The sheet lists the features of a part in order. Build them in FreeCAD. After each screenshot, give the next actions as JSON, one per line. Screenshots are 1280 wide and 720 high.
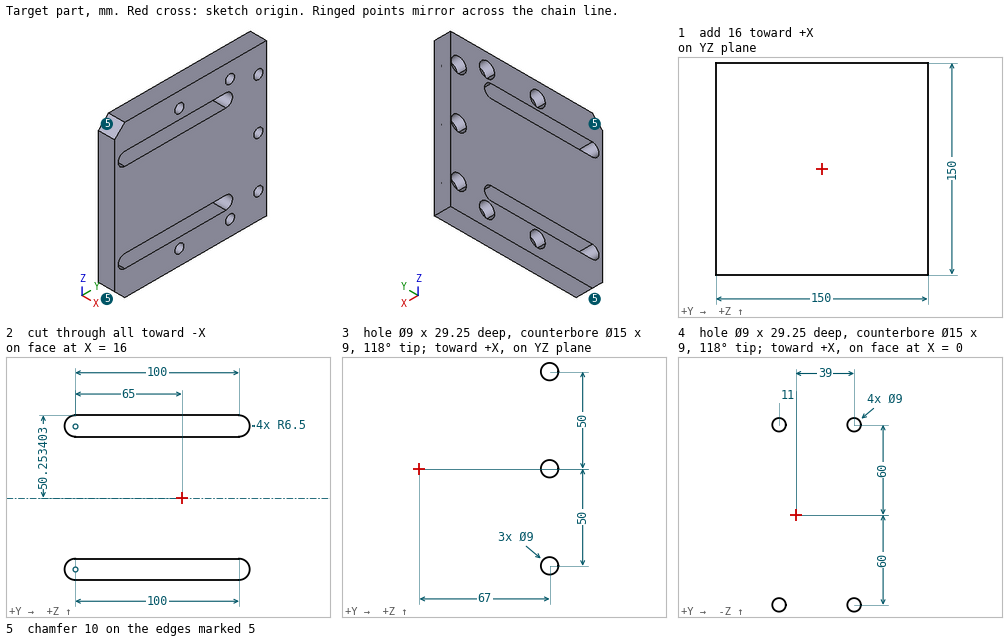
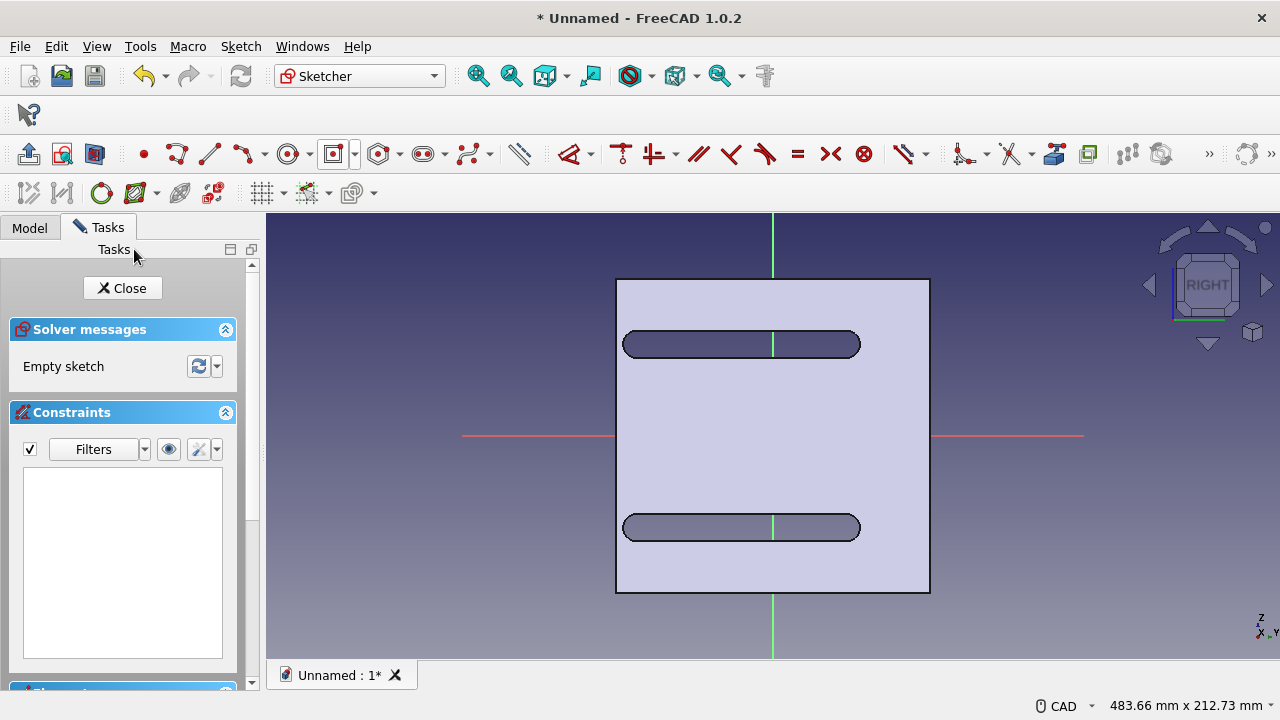
{"action": "left_click", "coordinate": [95, 154]}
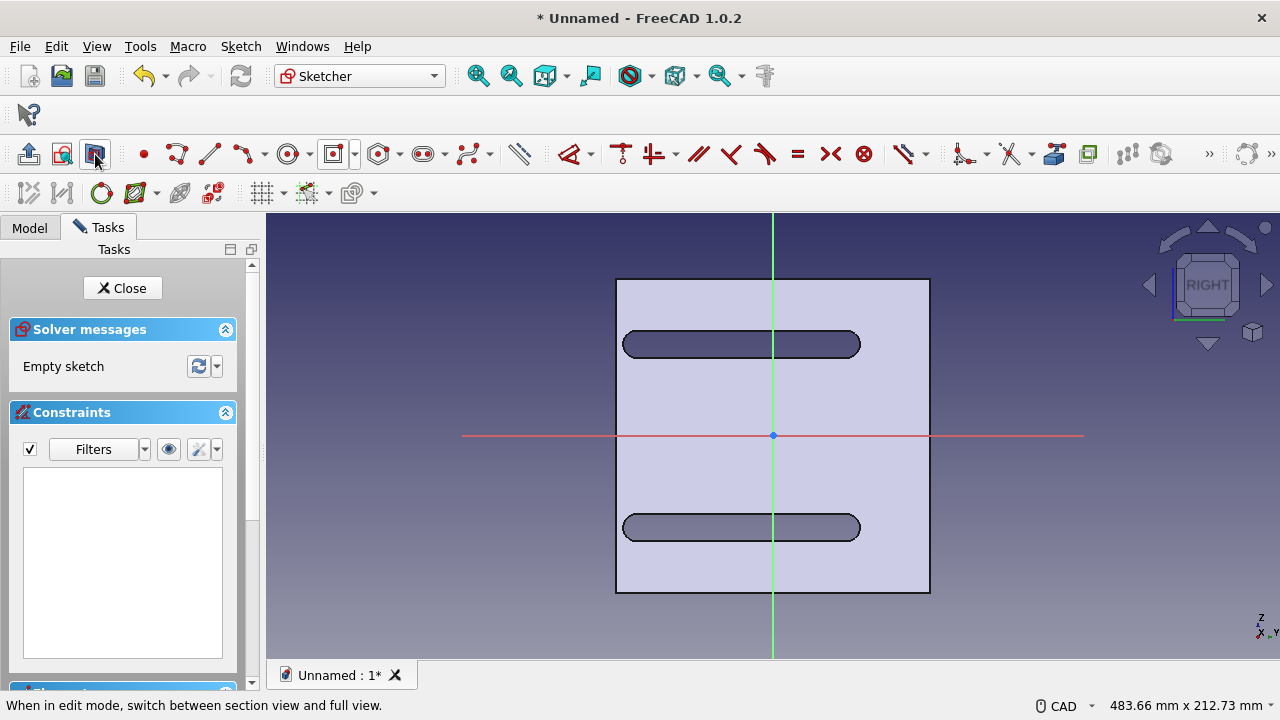
{"action": "key", "text": "g c"}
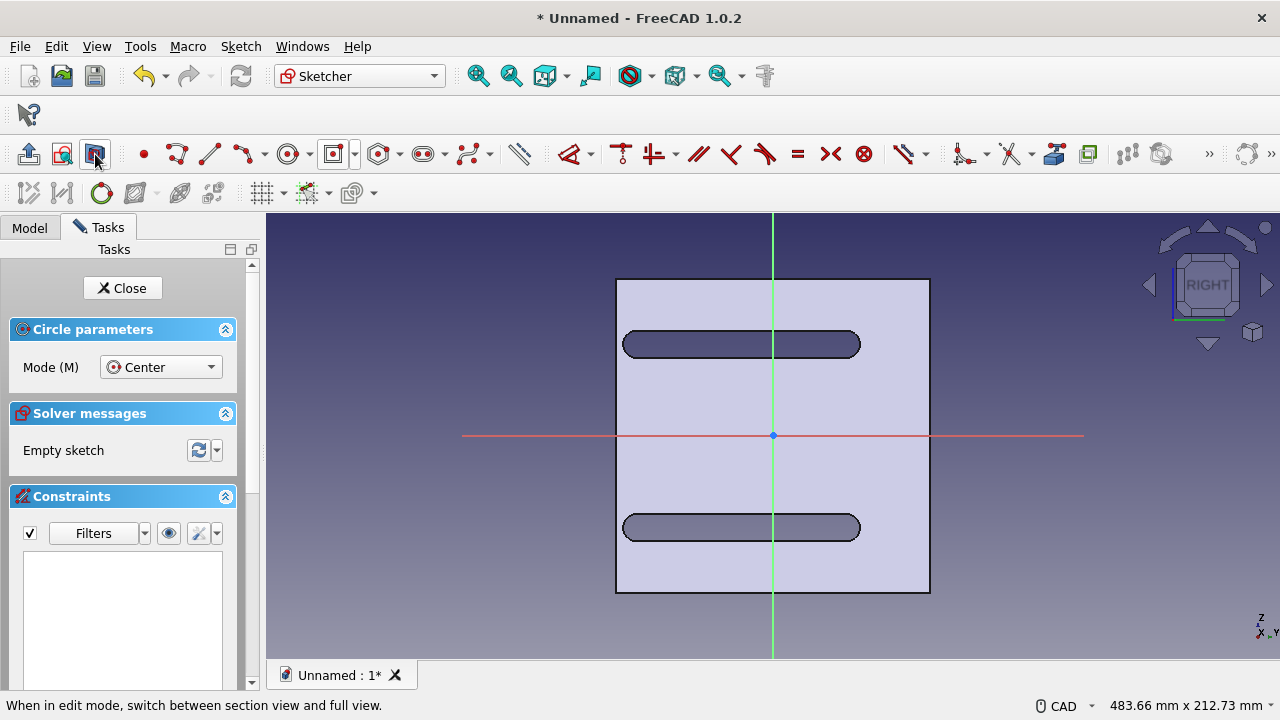
{"action": "scroll", "coordinate": [913, 541], "scroll_direction": "up", "scroll_amount": 5}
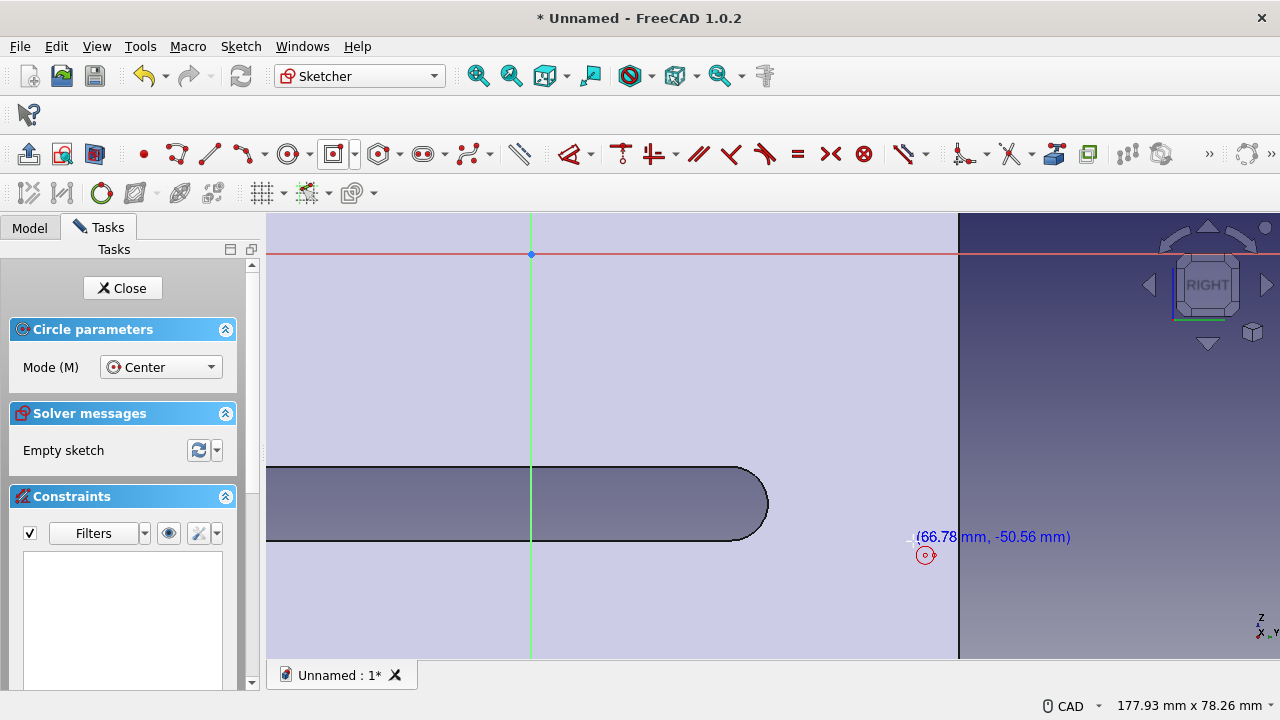
{"action": "left_click", "coordinate": [913, 539]}
{"action": "mouse_move", "coordinate": [931, 521]}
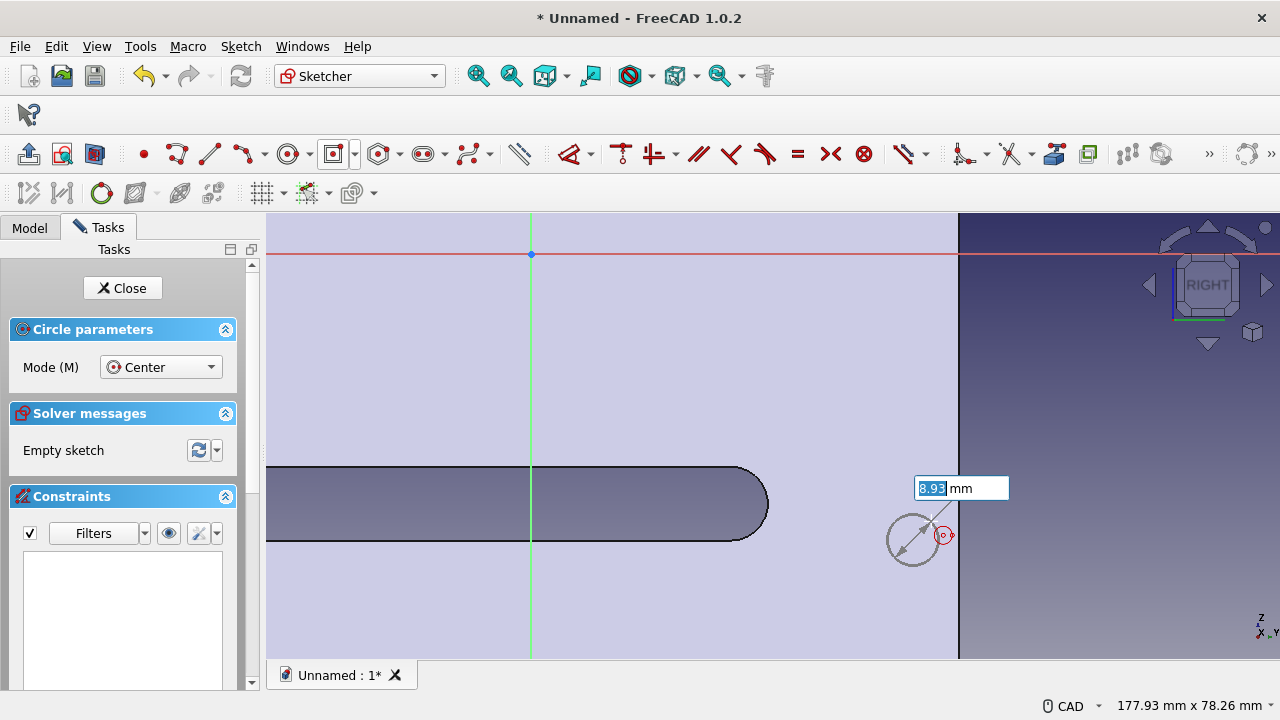
{"action": "type", "text": "9"}
{"action": "key", "text": "Return"}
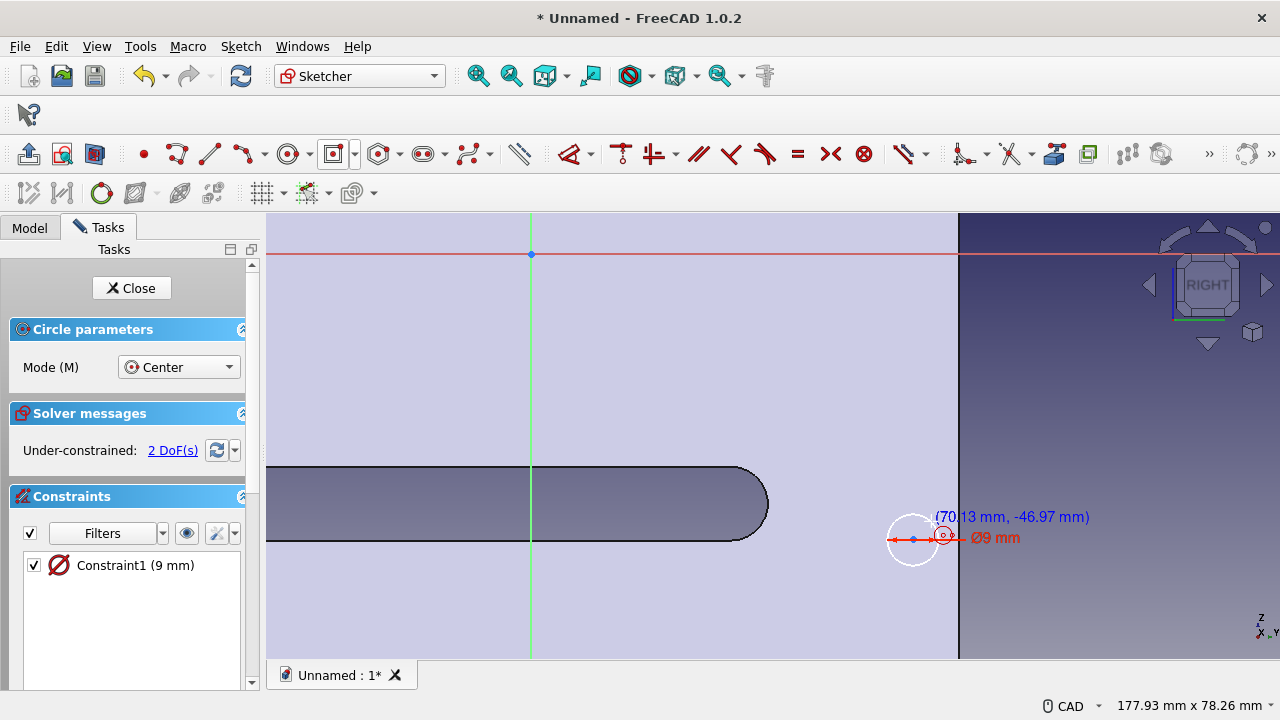
{"action": "left_click", "coordinate": [913, 254]}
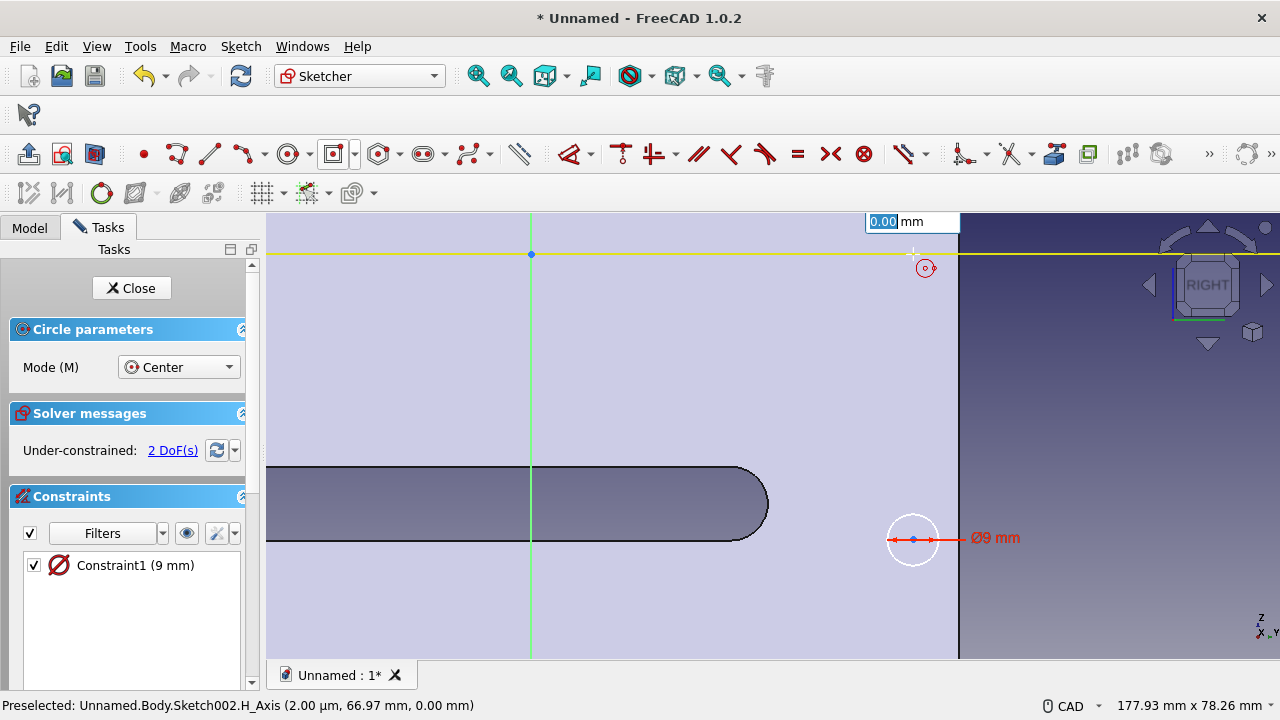
{"action": "scroll", "coordinate": [680, 584], "scroll_direction": "down", "scroll_amount": 4}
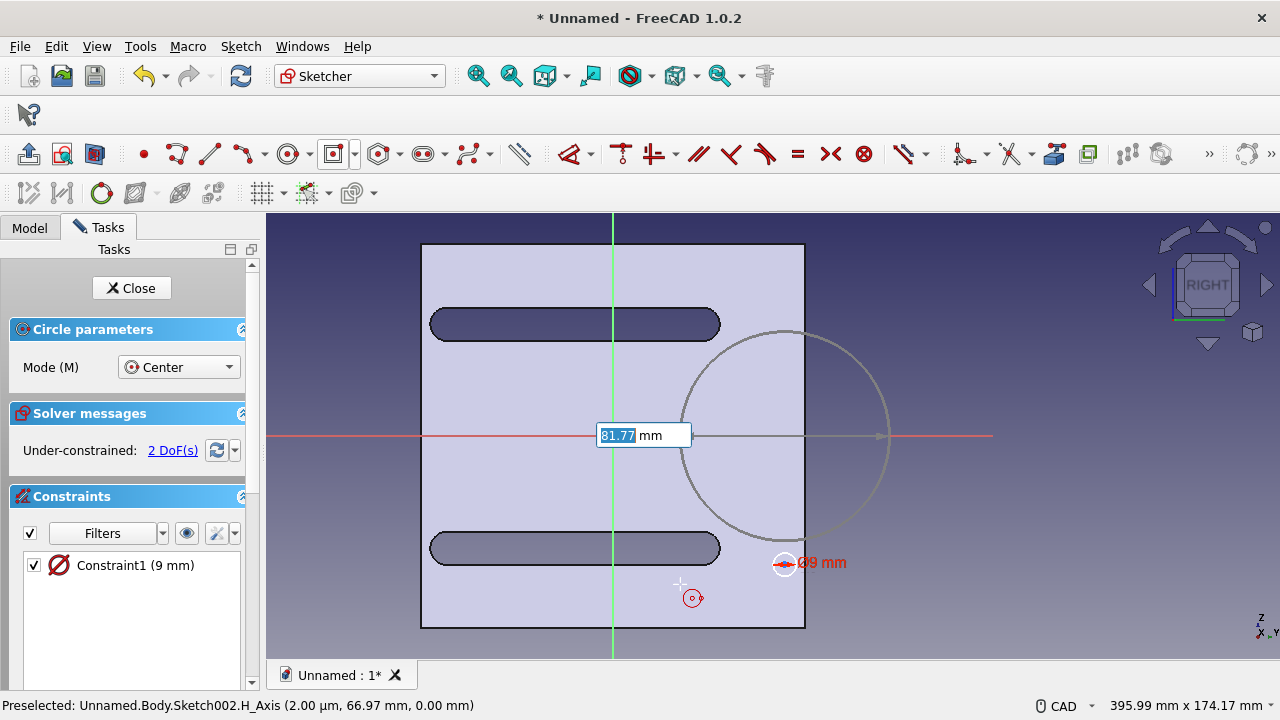
{"action": "scroll", "coordinate": [793, 428], "scroll_direction": "up", "scroll_amount": 4}
{"action": "mouse_move", "coordinate": [793, 428]}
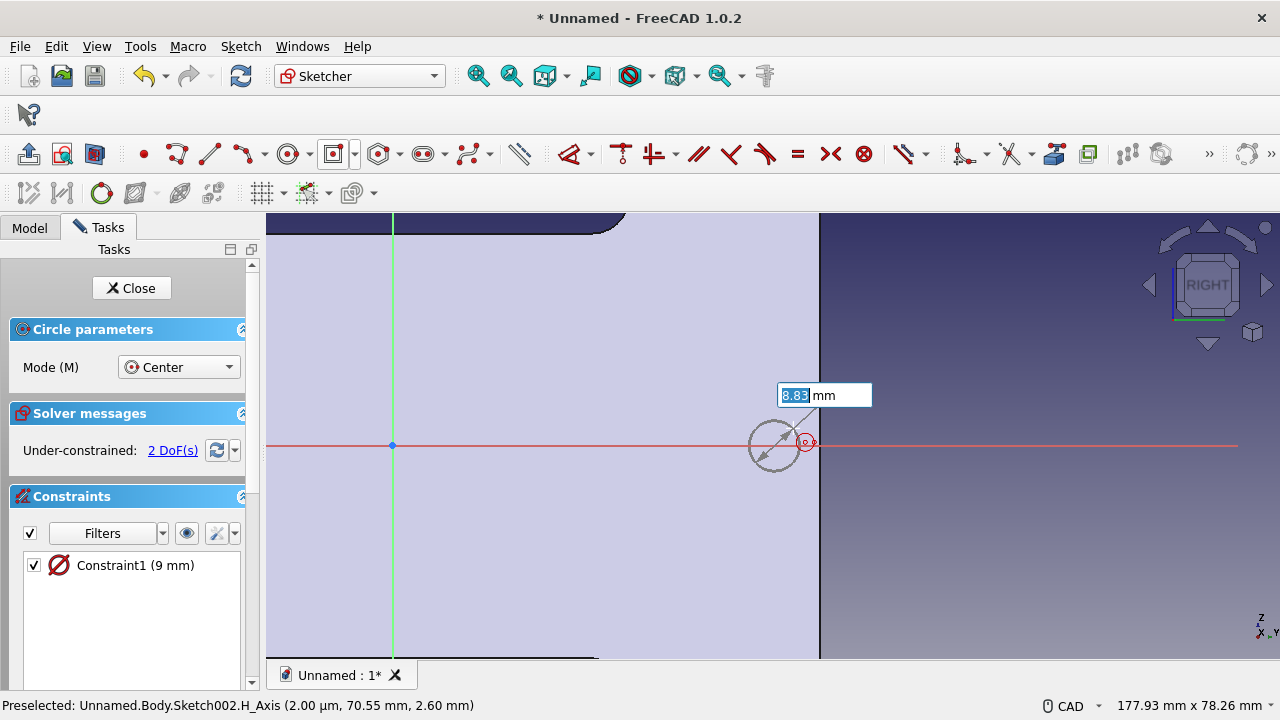
{"action": "type", "text": "9"}
{"action": "key", "text": "Return"}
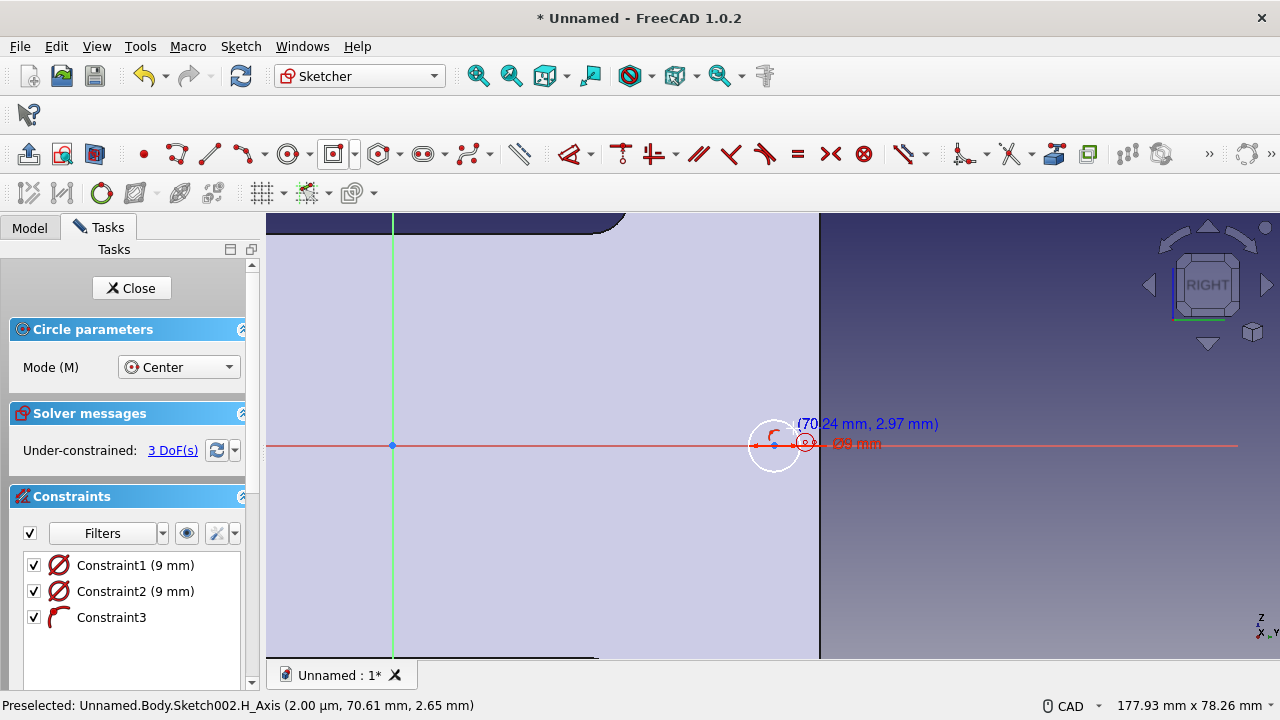
{"action": "scroll", "coordinate": [793, 428], "scroll_direction": "down", "scroll_amount": 4}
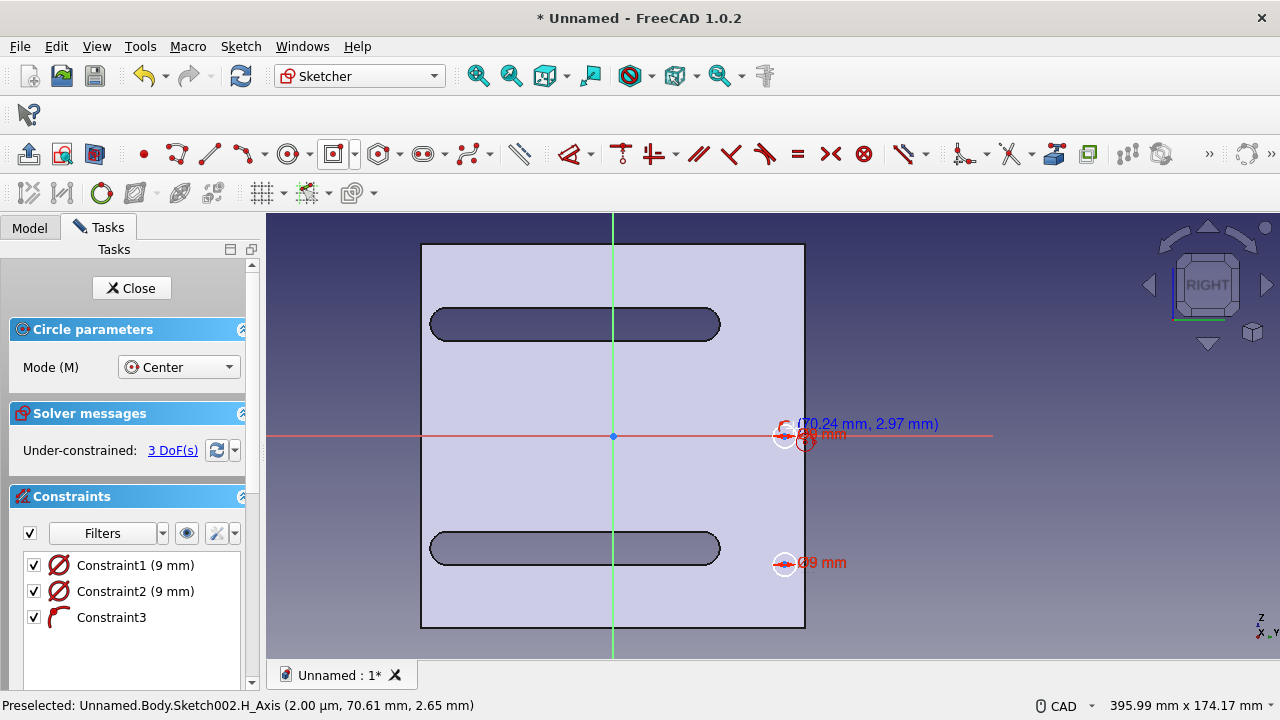
{"action": "scroll", "coordinate": [785, 308], "scroll_direction": "up", "scroll_amount": 4}